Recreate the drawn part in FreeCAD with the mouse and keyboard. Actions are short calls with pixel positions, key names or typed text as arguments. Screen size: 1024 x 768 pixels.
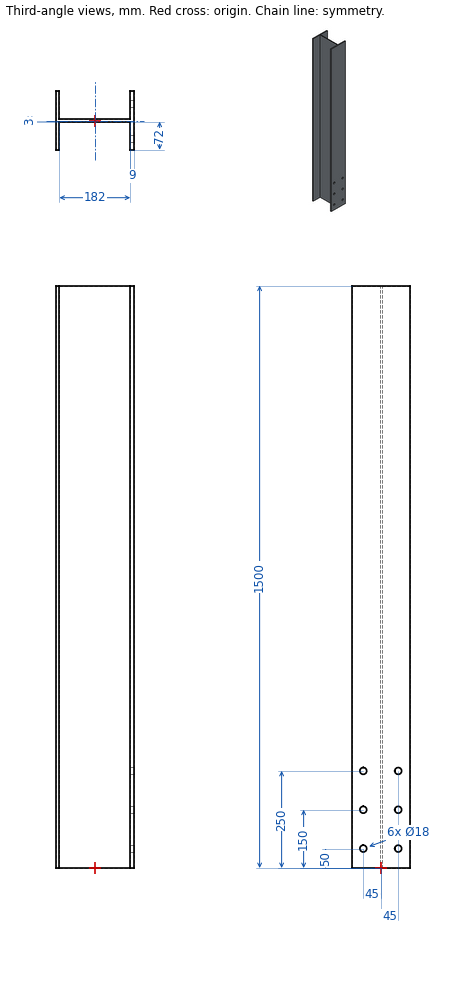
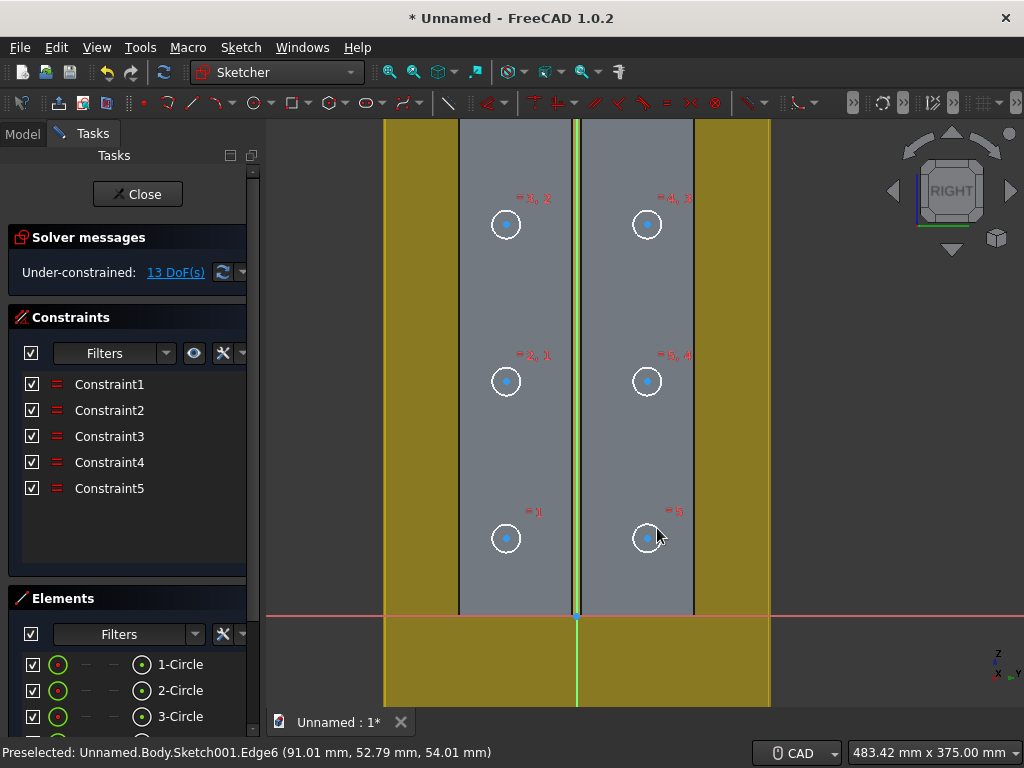
click(506, 539)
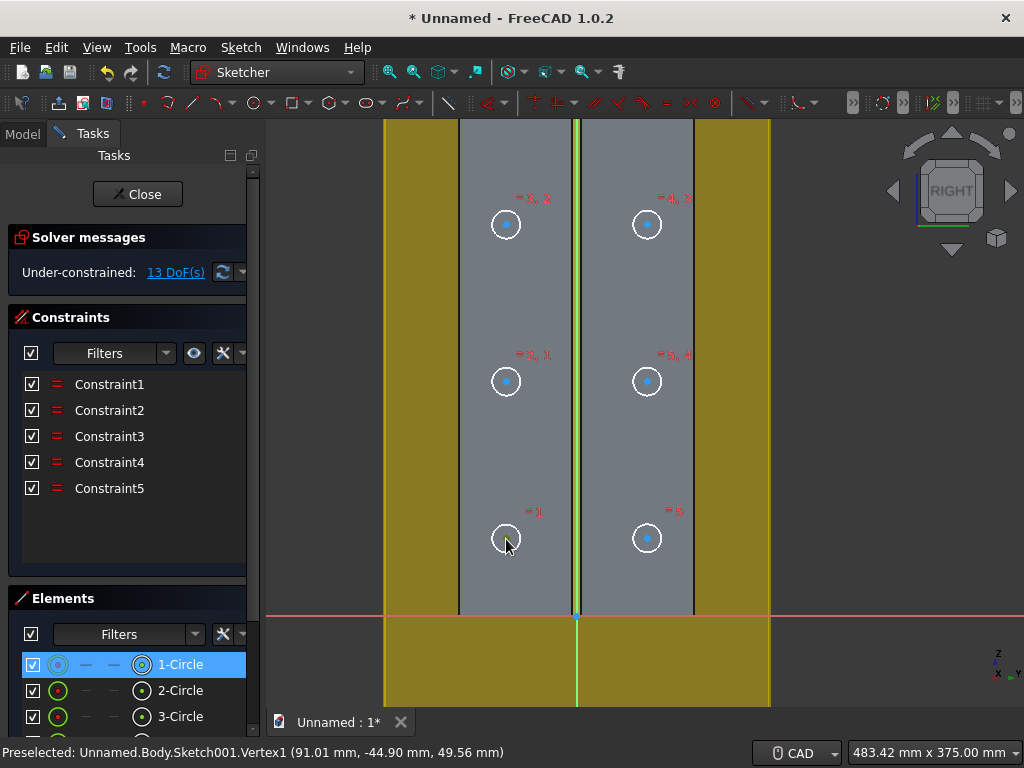
click(506, 382)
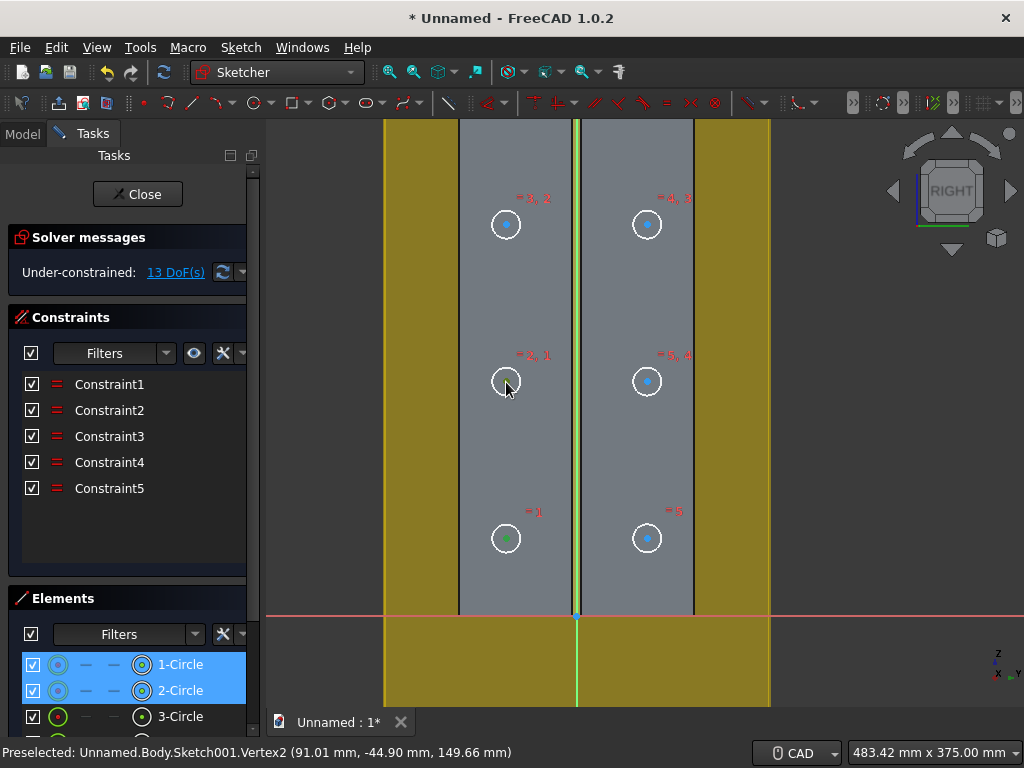
click(576, 104)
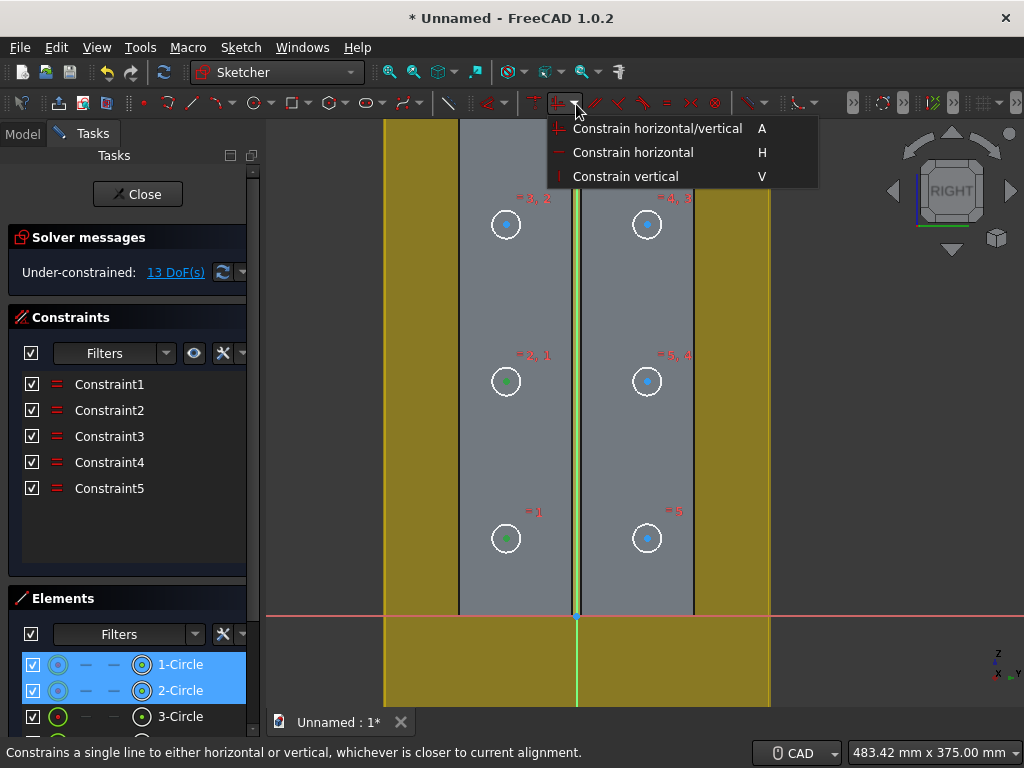
click(683, 176)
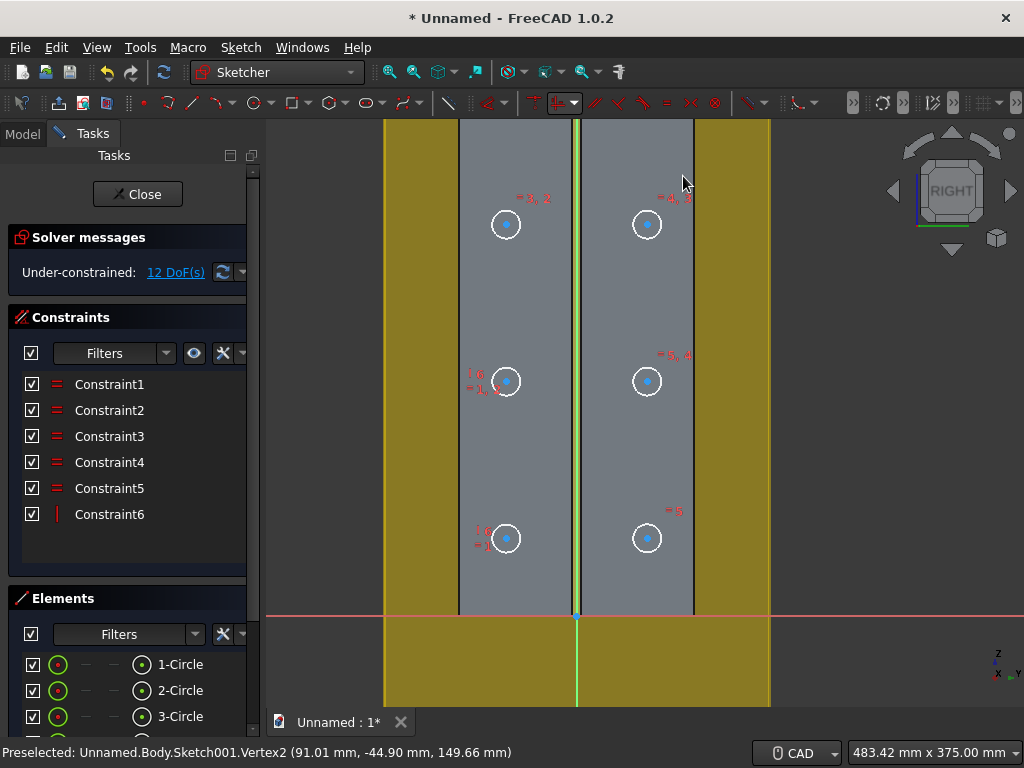
click(506, 382)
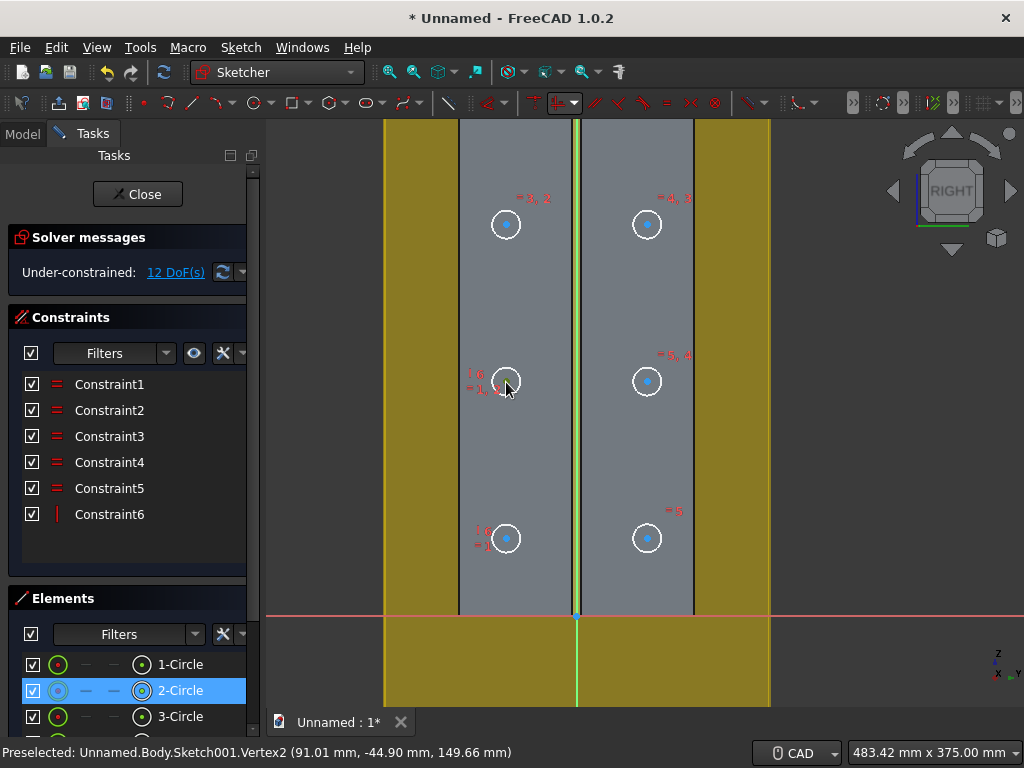
click(506, 225)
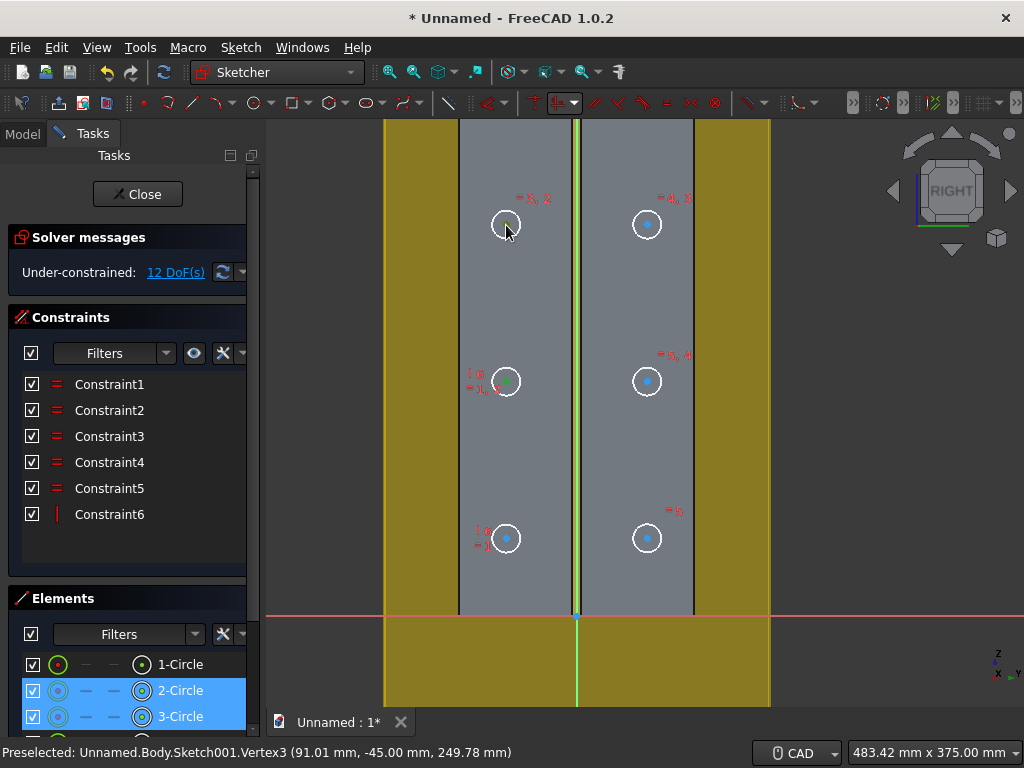
click(576, 104)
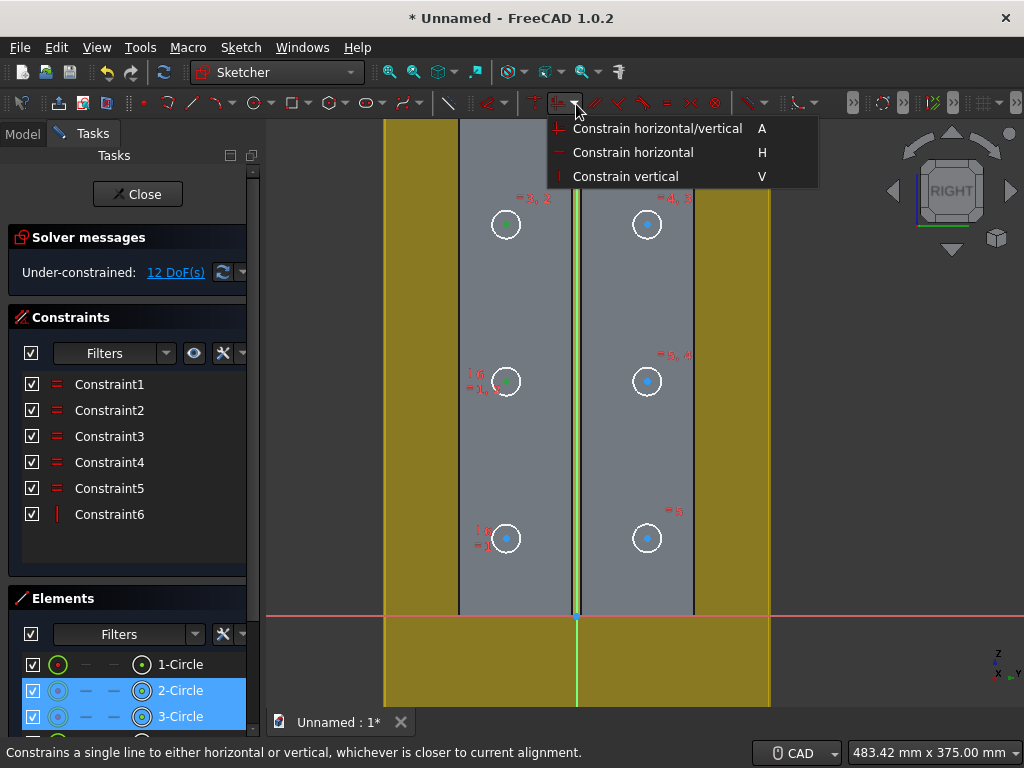
click(683, 176)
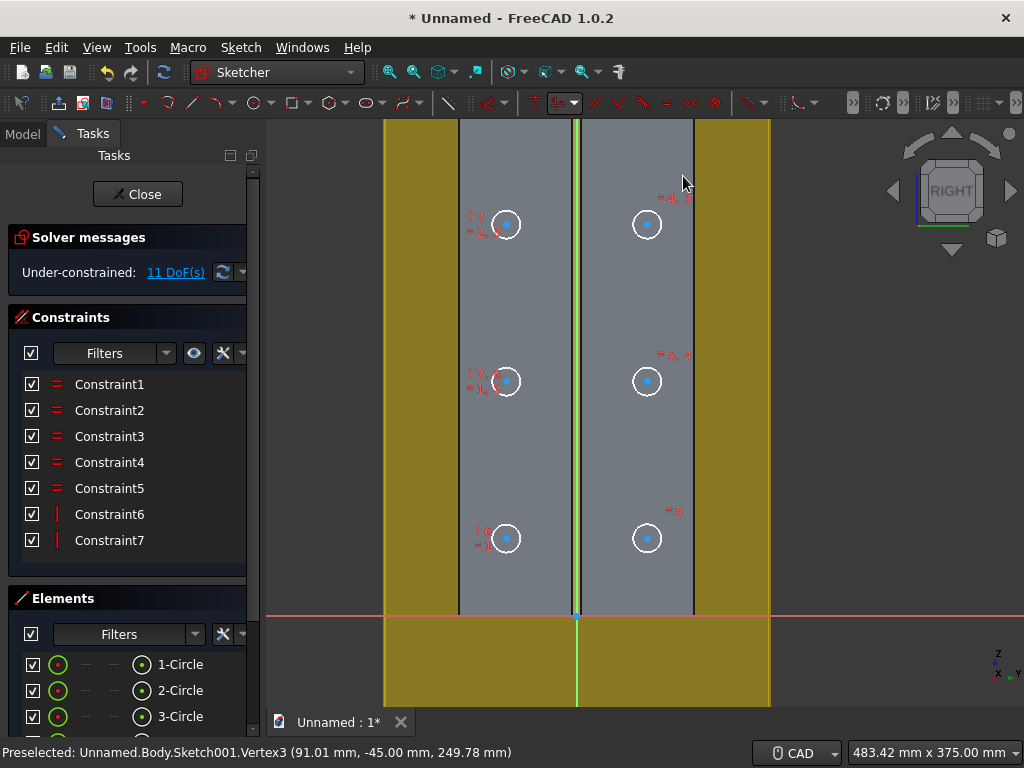
click(506, 225)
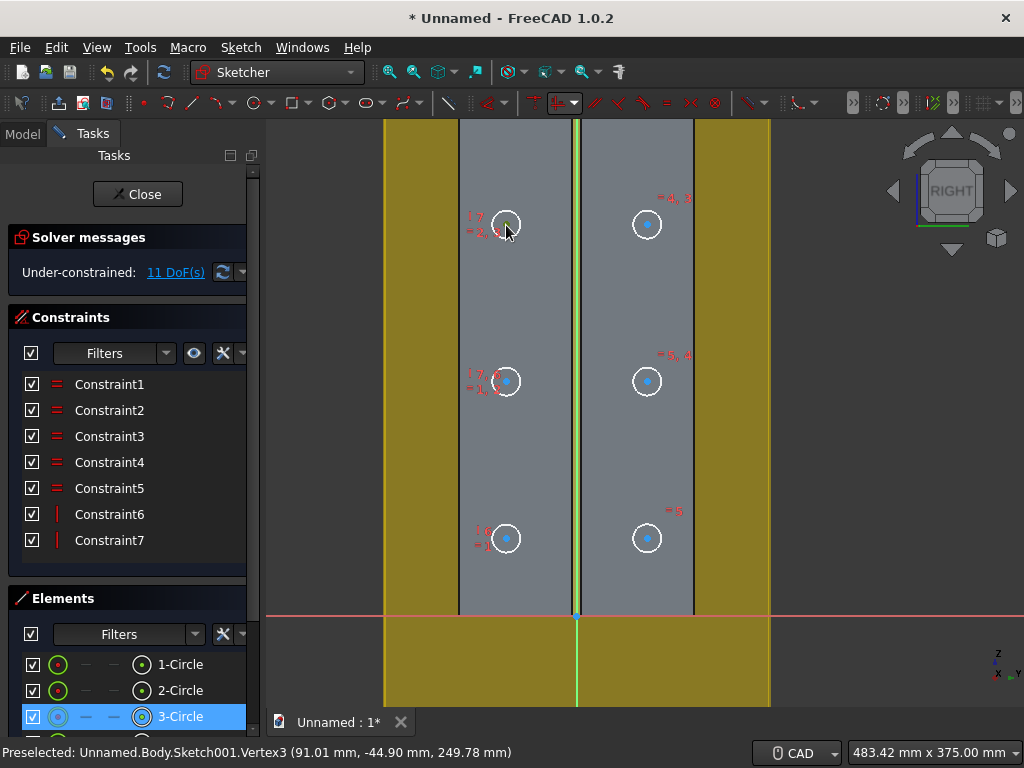
click(647, 225)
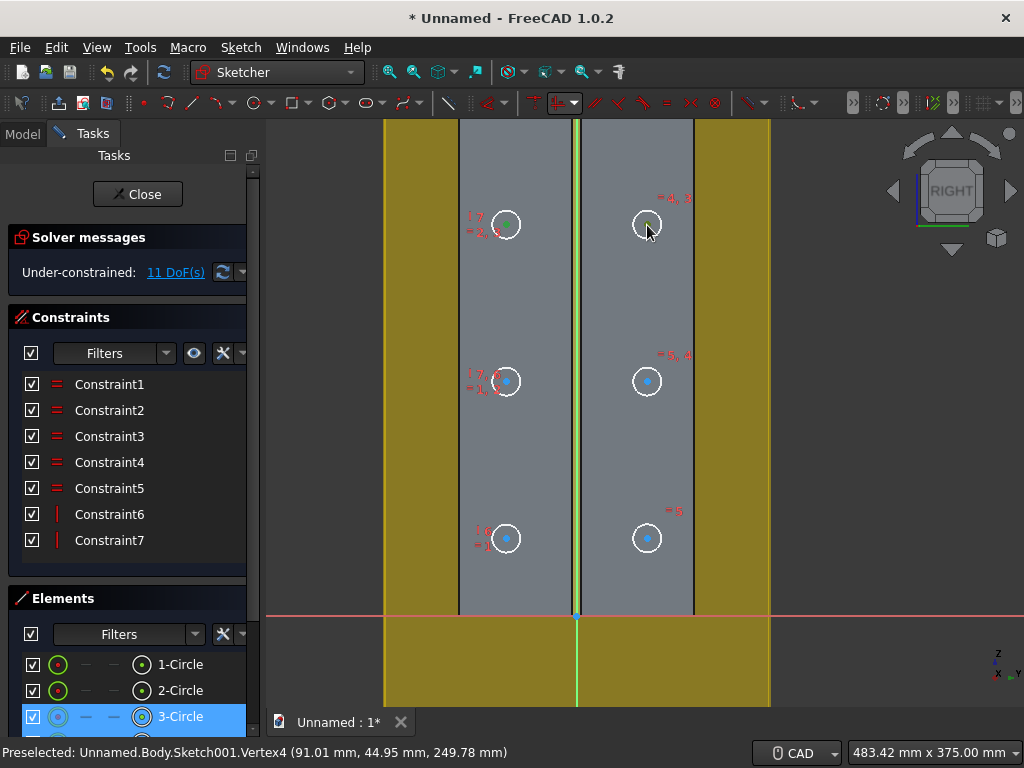
key(h)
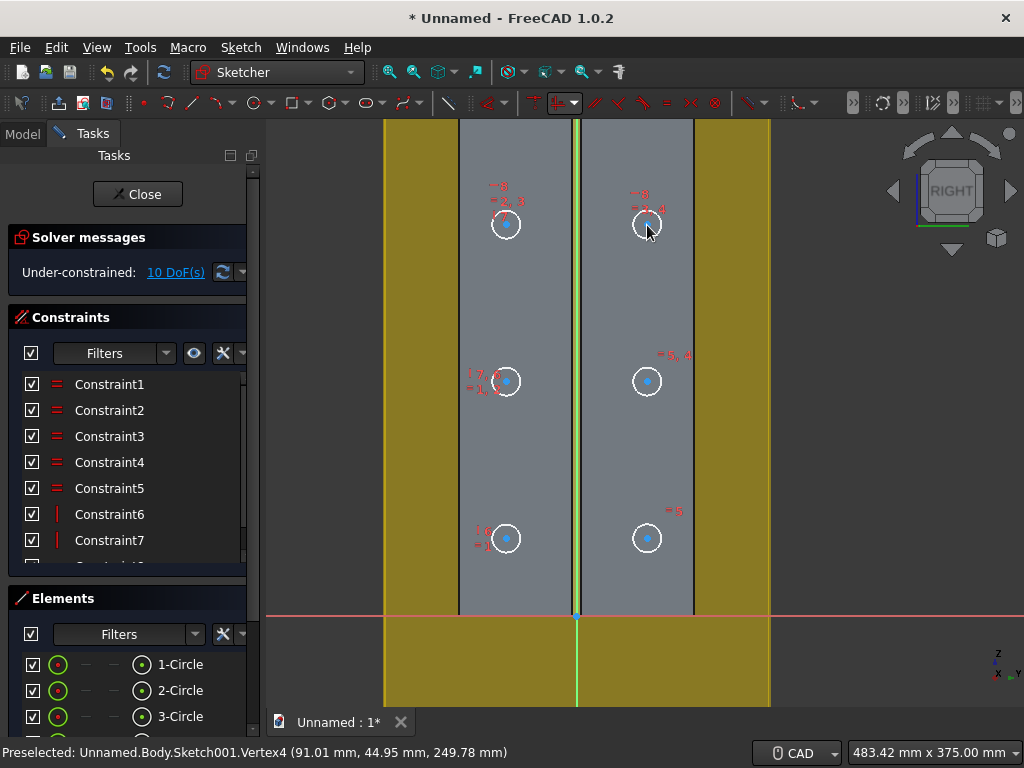
click(647, 225)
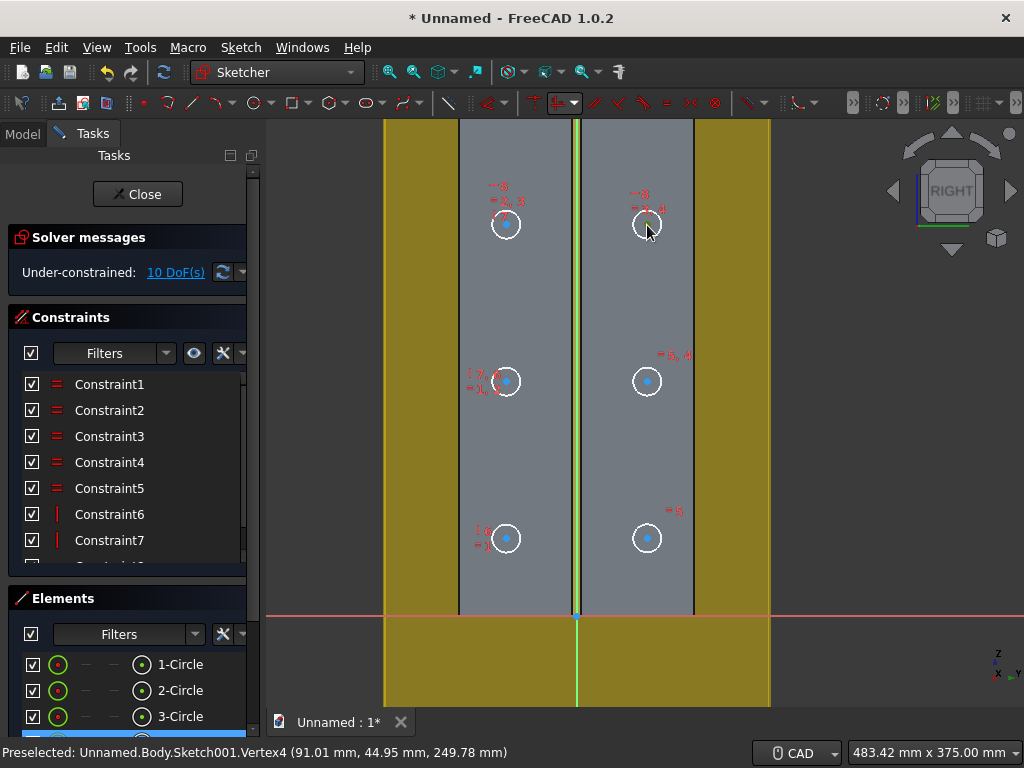
click(647, 382)